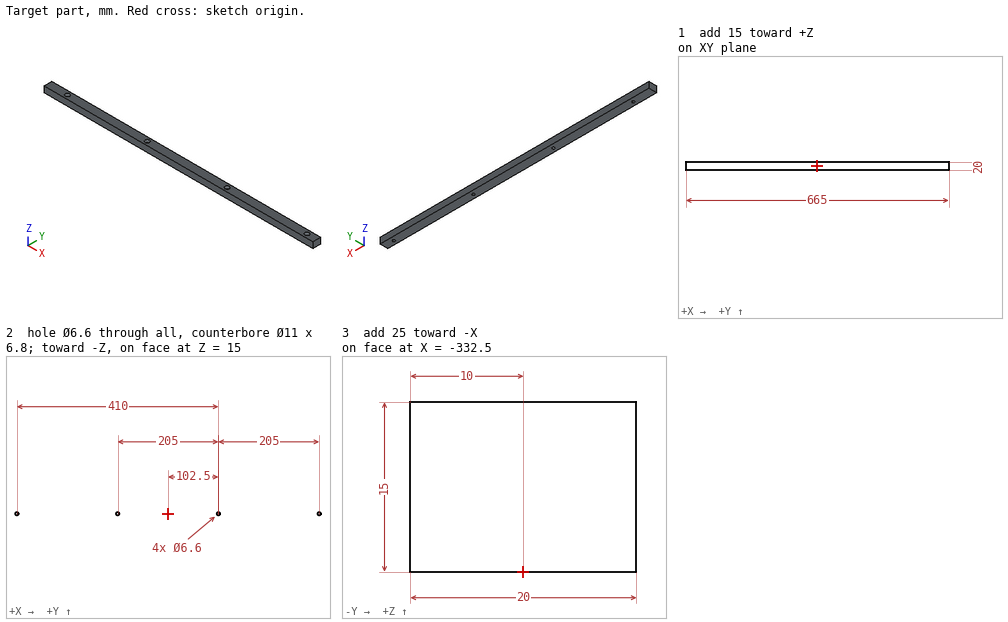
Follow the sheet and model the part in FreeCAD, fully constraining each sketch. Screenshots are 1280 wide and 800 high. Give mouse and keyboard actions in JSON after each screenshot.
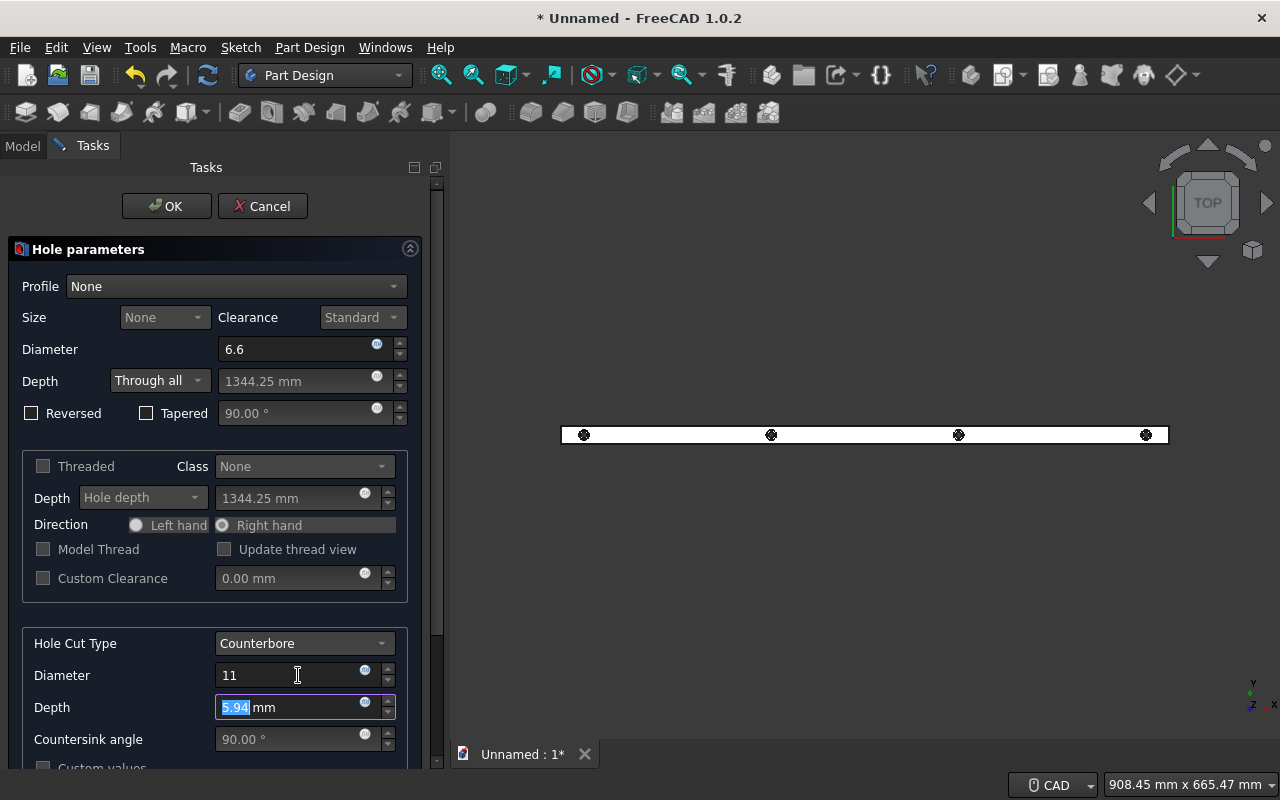
{"action": "type", "text": "6.8"}
{"action": "key", "text": "Tab"}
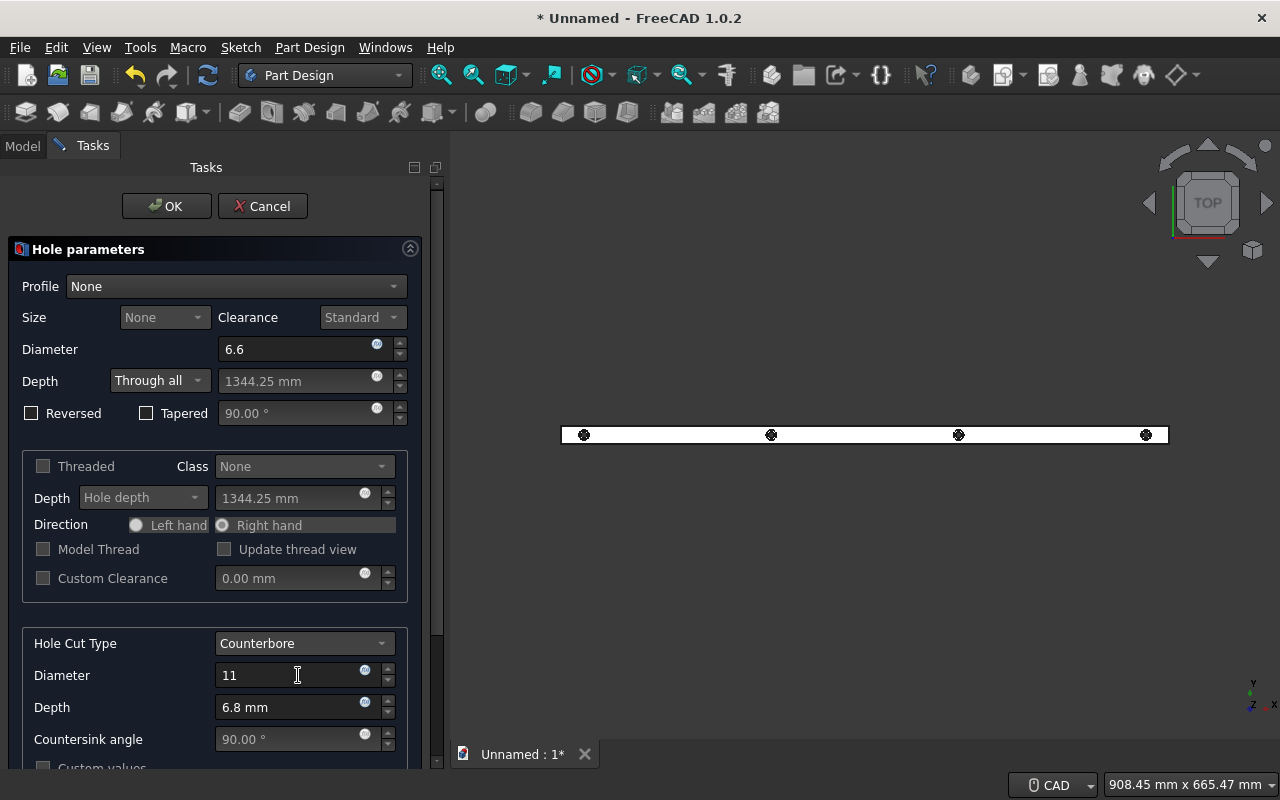
{"action": "left_click", "coordinate": [167, 206]}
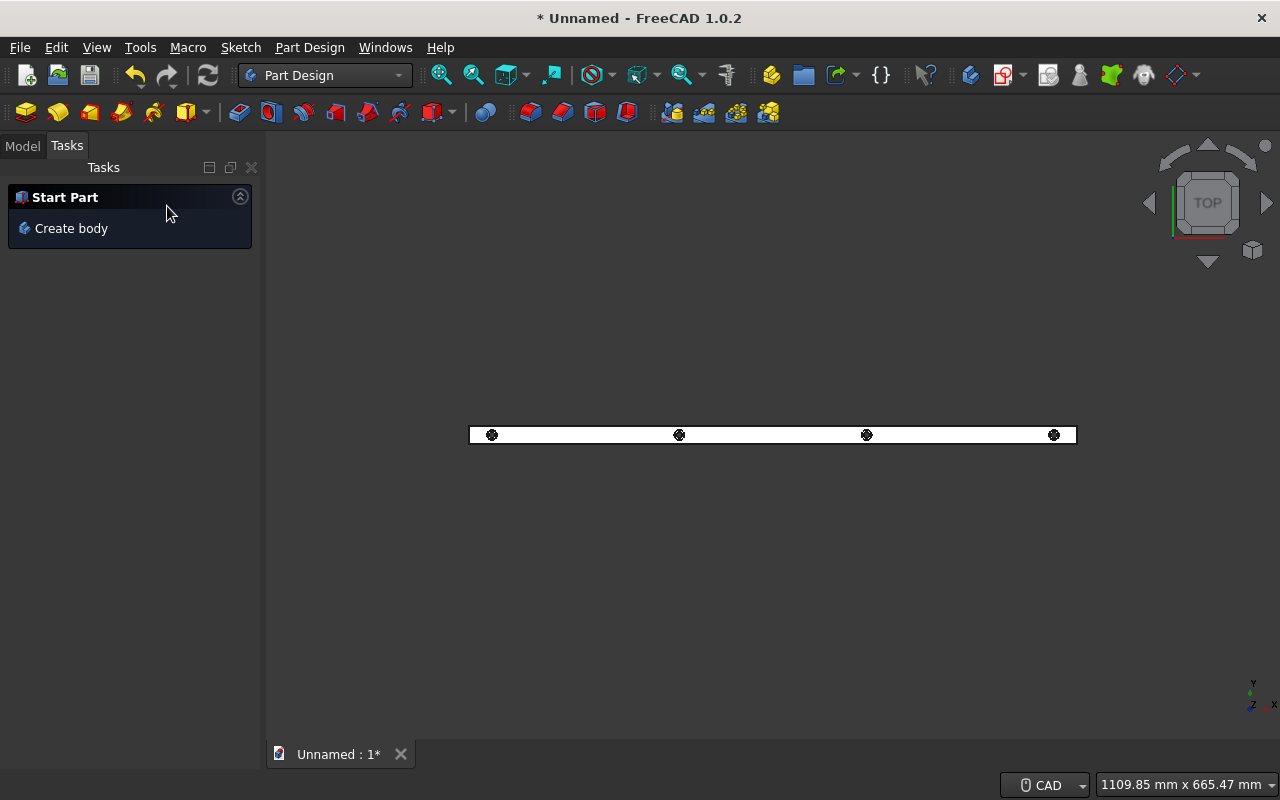
{"action": "key", "text": "6"}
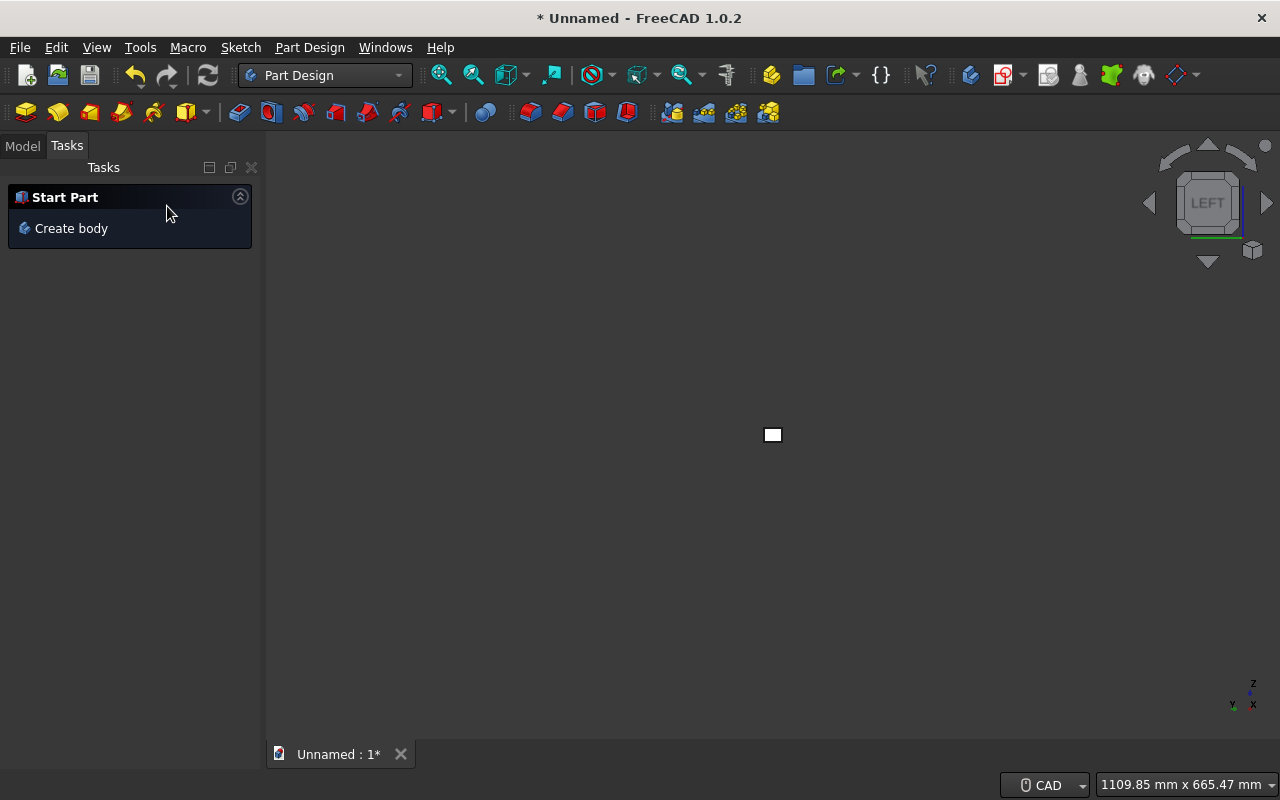
{"action": "key", "text": "v f"}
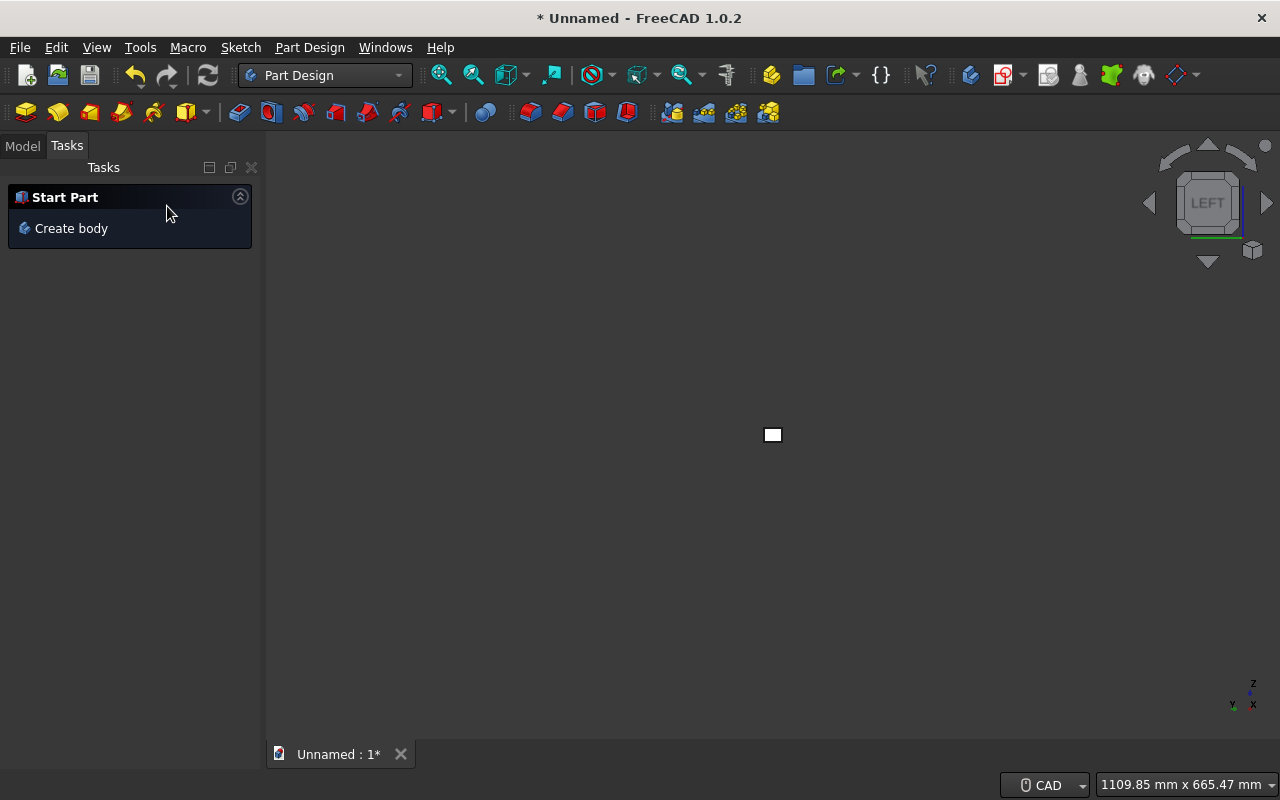
{"action": "scroll", "coordinate": [773, 434], "scroll_direction": "up", "scroll_amount": 3}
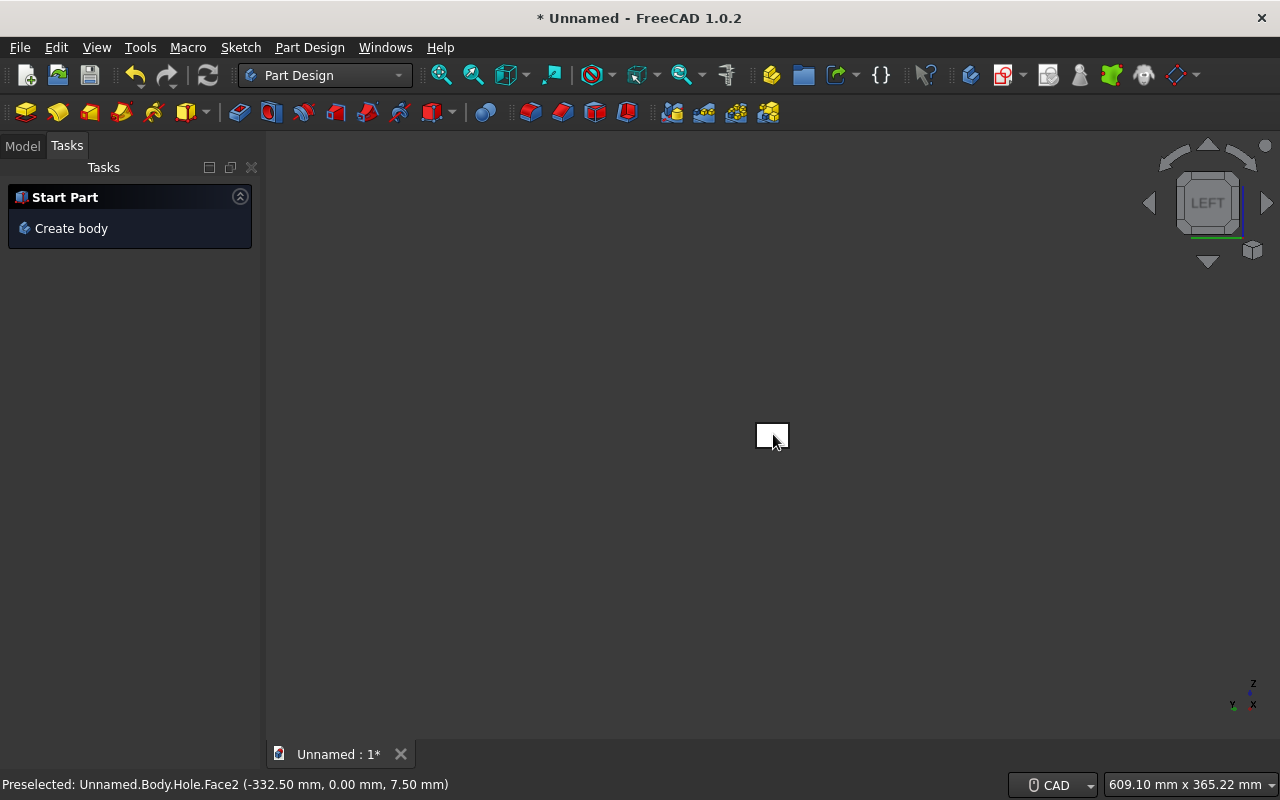
{"action": "left_click", "coordinate": [773, 434]}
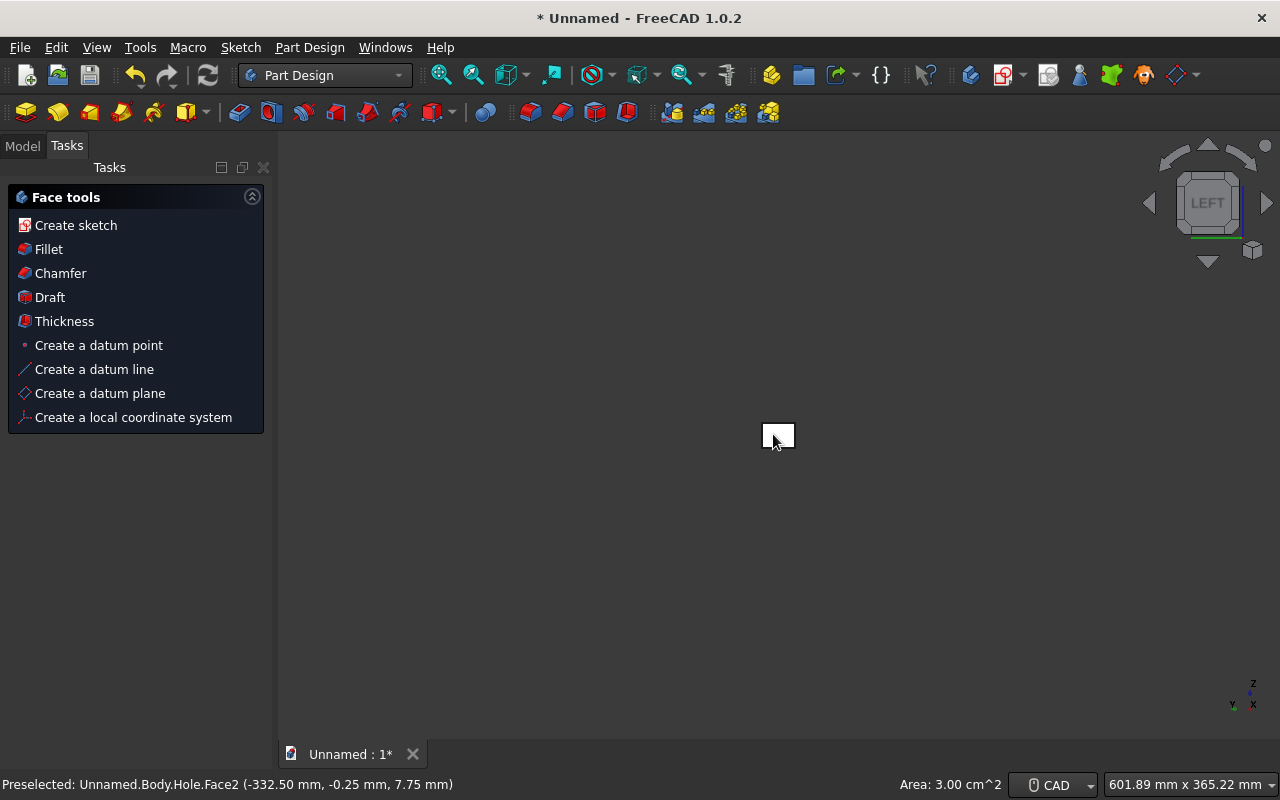
{"action": "left_click", "coordinate": [1004, 76]}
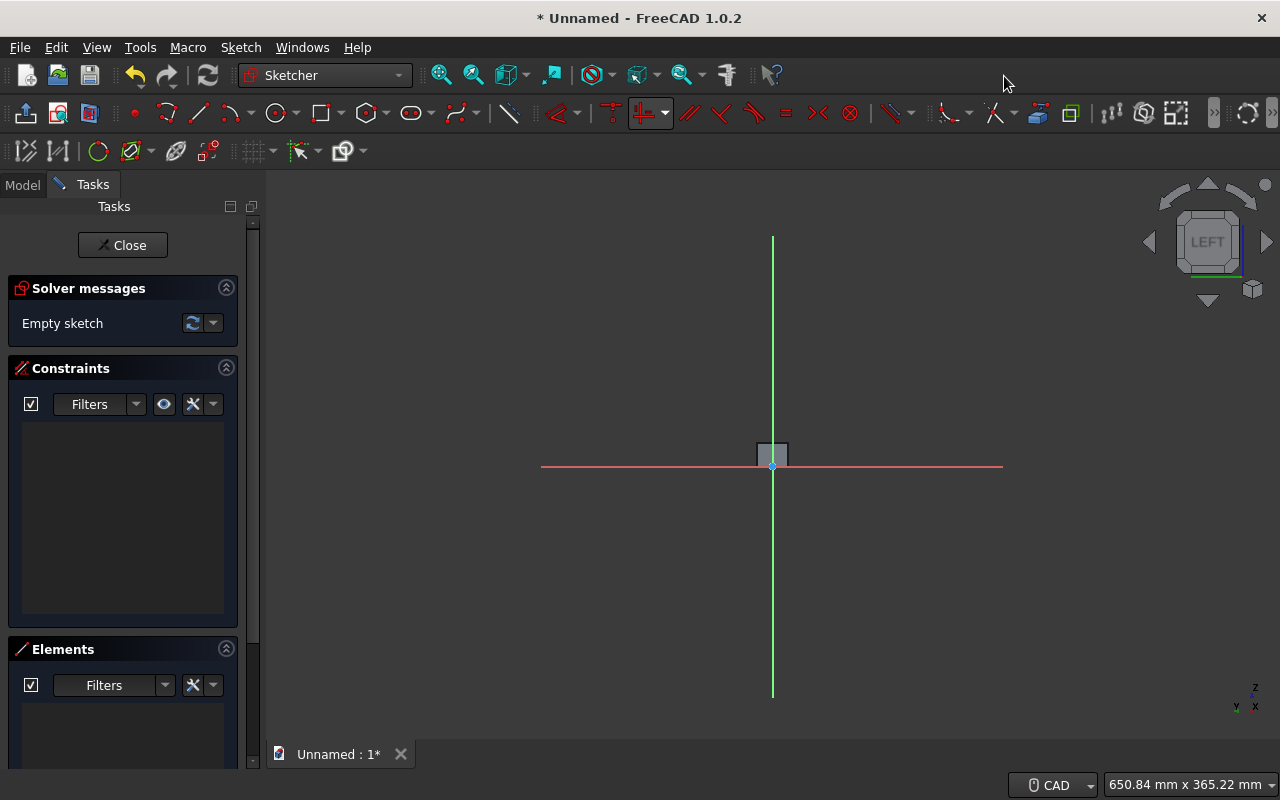
{"action": "scroll", "coordinate": [777, 455], "scroll_direction": "up", "scroll_amount": 14}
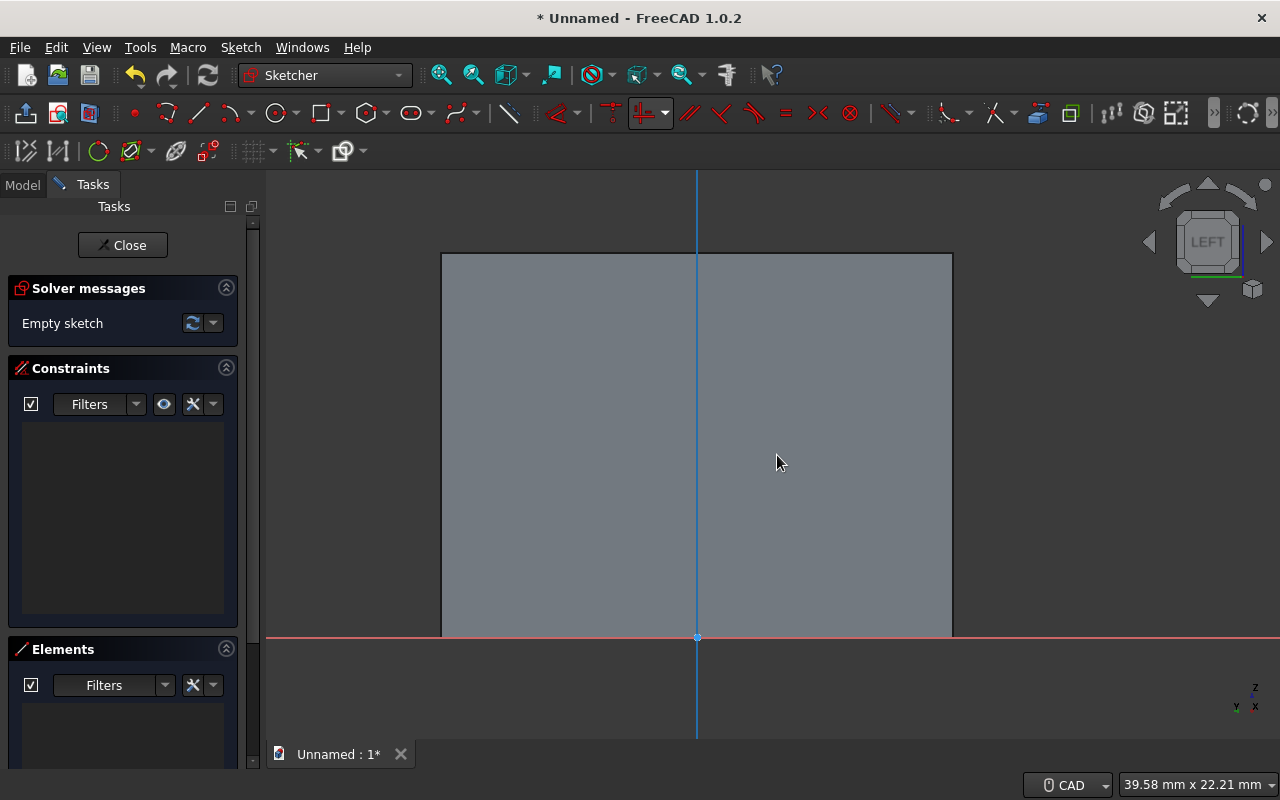
{"action": "key", "text": "g r"}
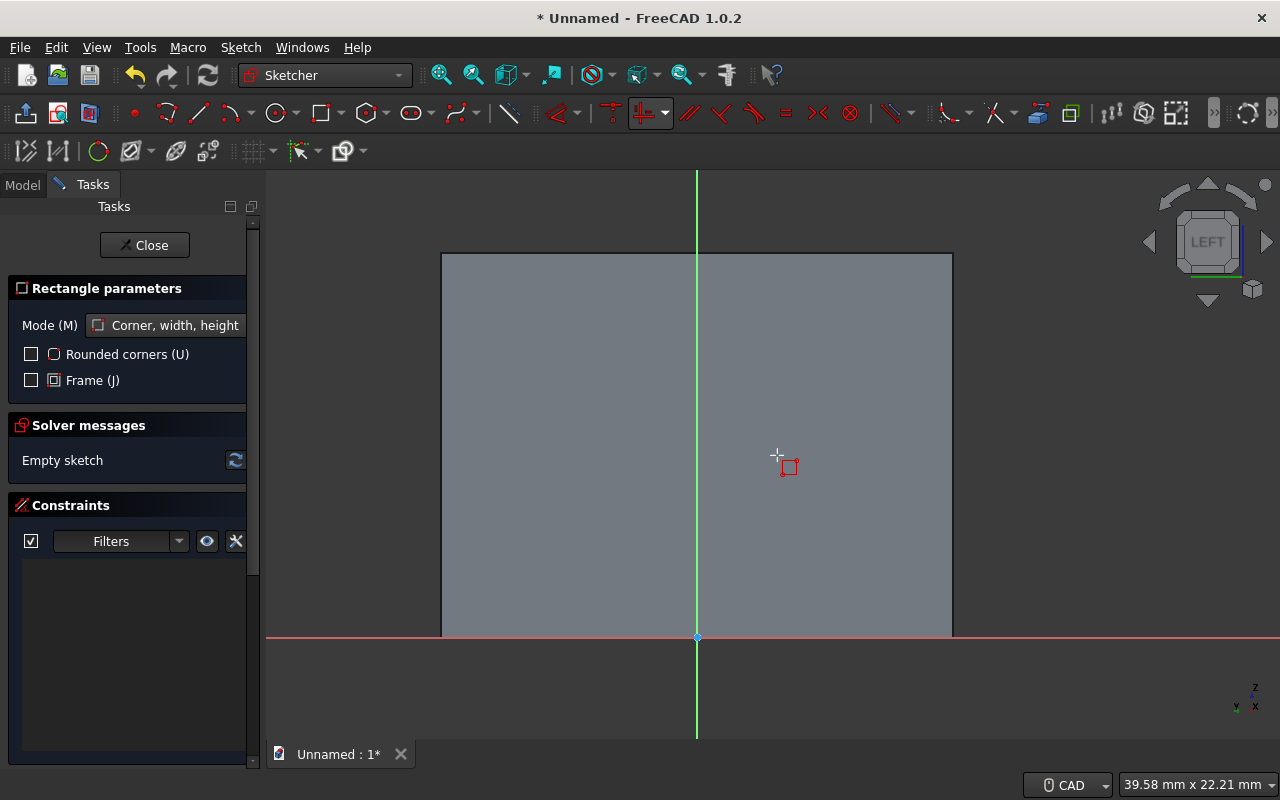
{"action": "left_click", "coordinate": [441, 253]}
{"action": "left_click", "coordinate": [953, 638]}
{"action": "key", "text": "Escape"}